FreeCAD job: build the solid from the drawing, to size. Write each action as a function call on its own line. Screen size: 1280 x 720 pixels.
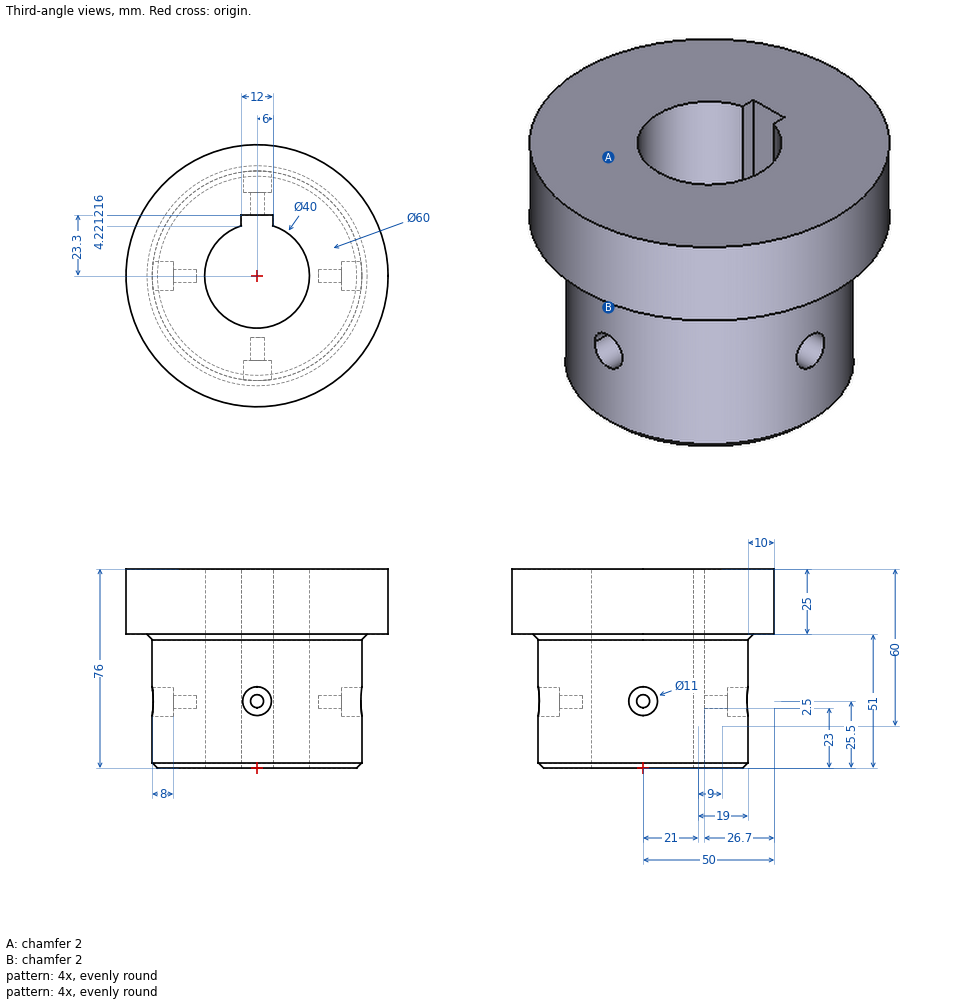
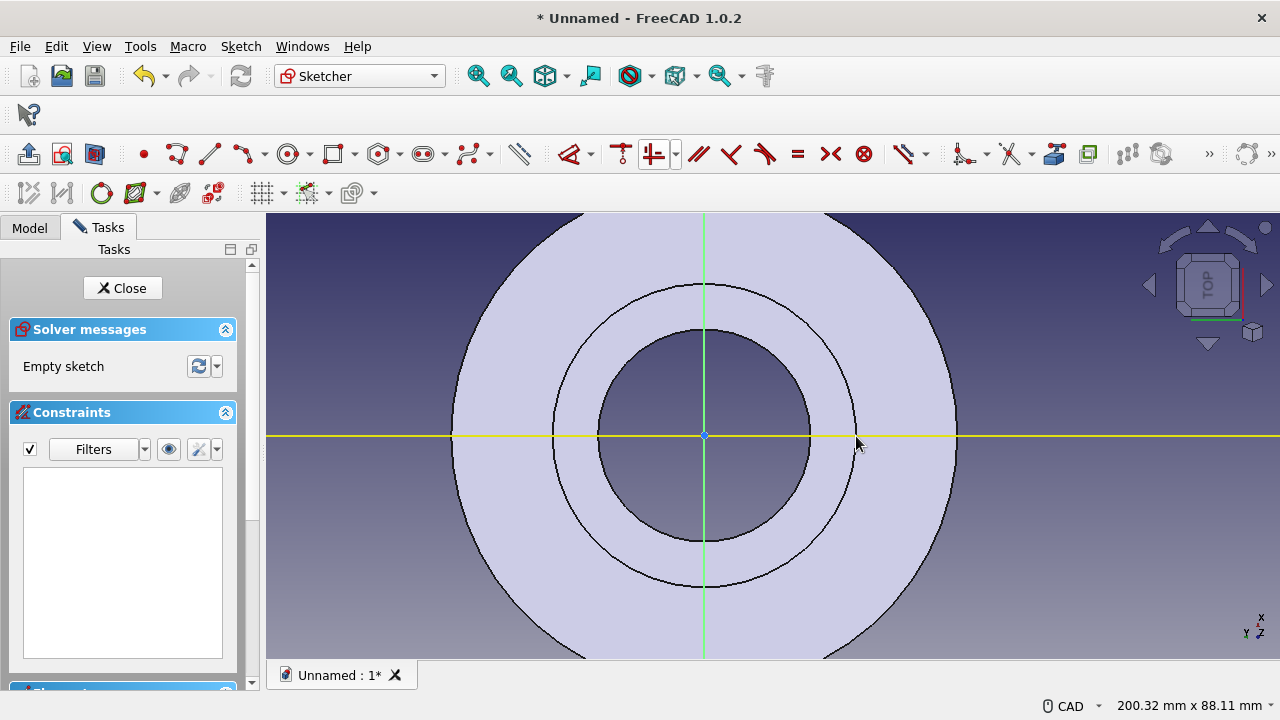
key(g)
key(c)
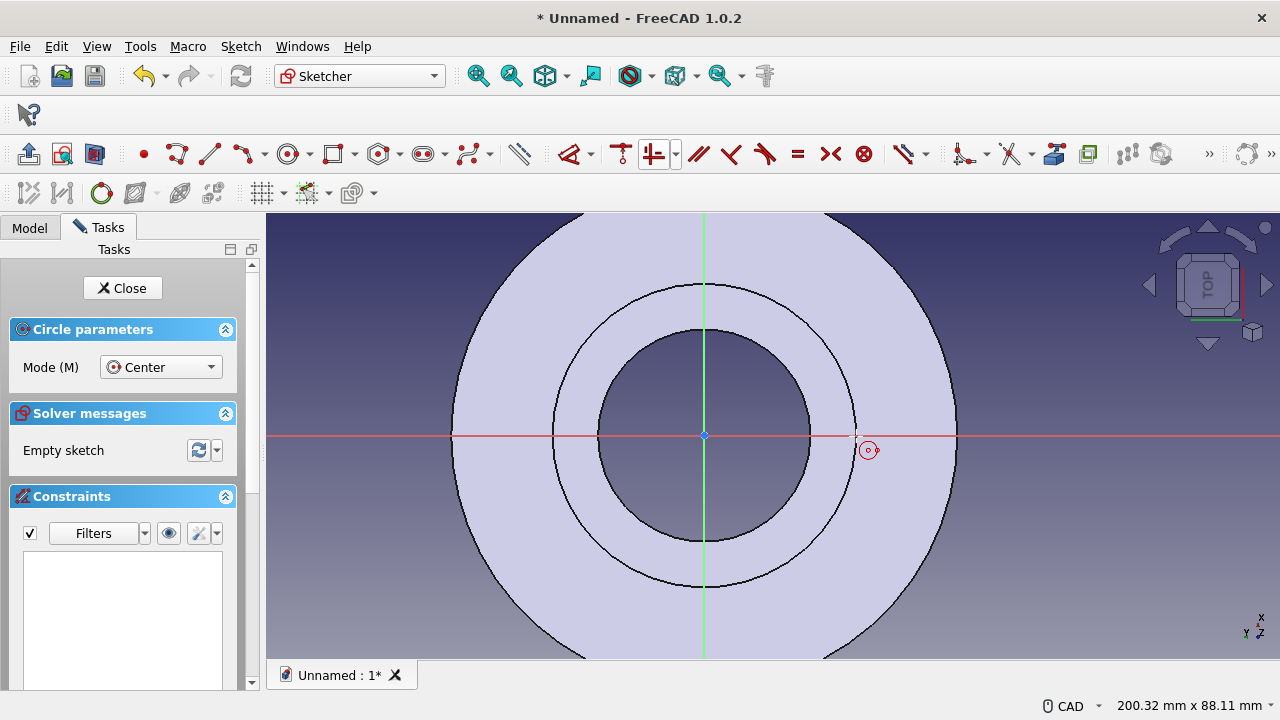
click(704, 436)
move(812, 328)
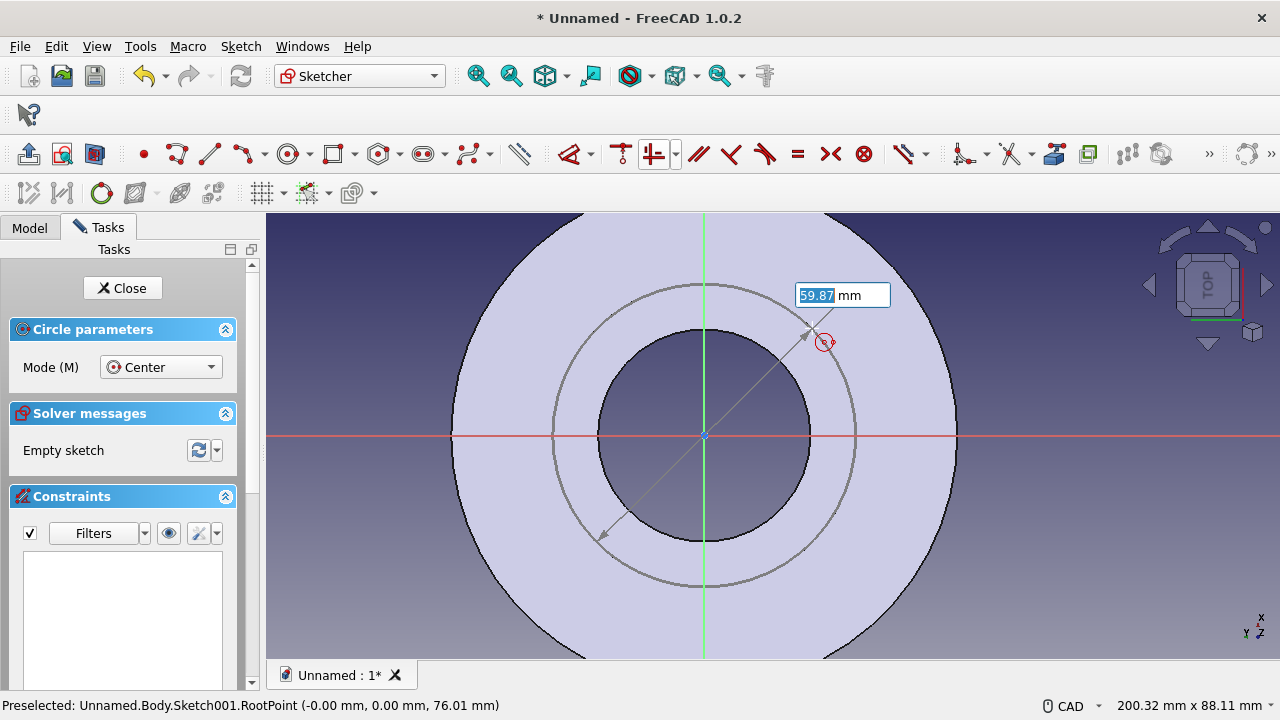
text(60)
key(Return)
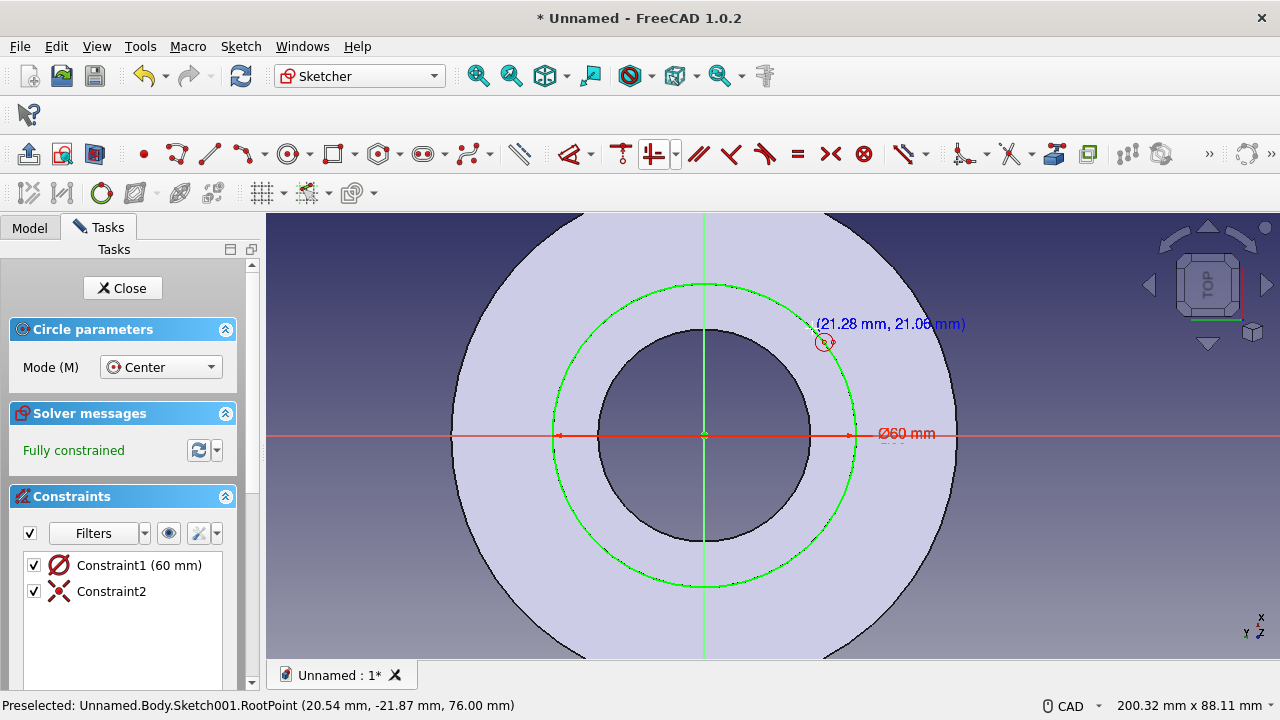
click(704, 436)
move(776, 364)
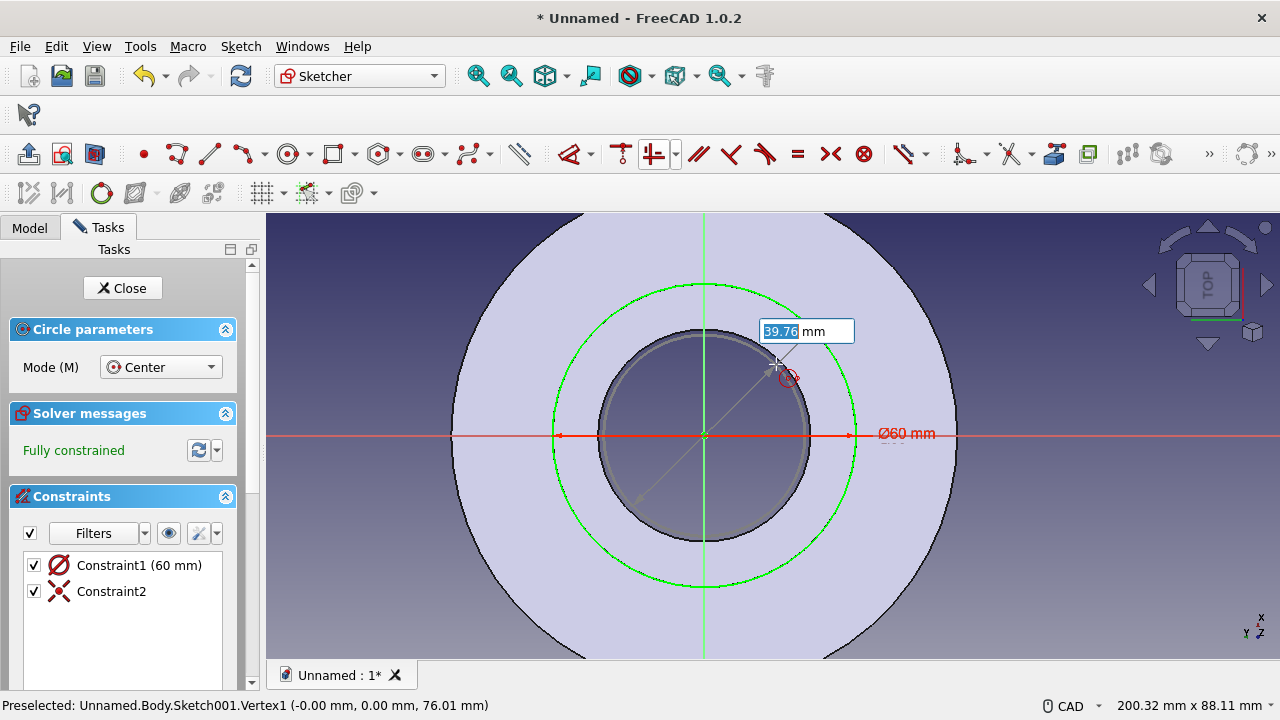
text(40)
key(Return)
key(Escape)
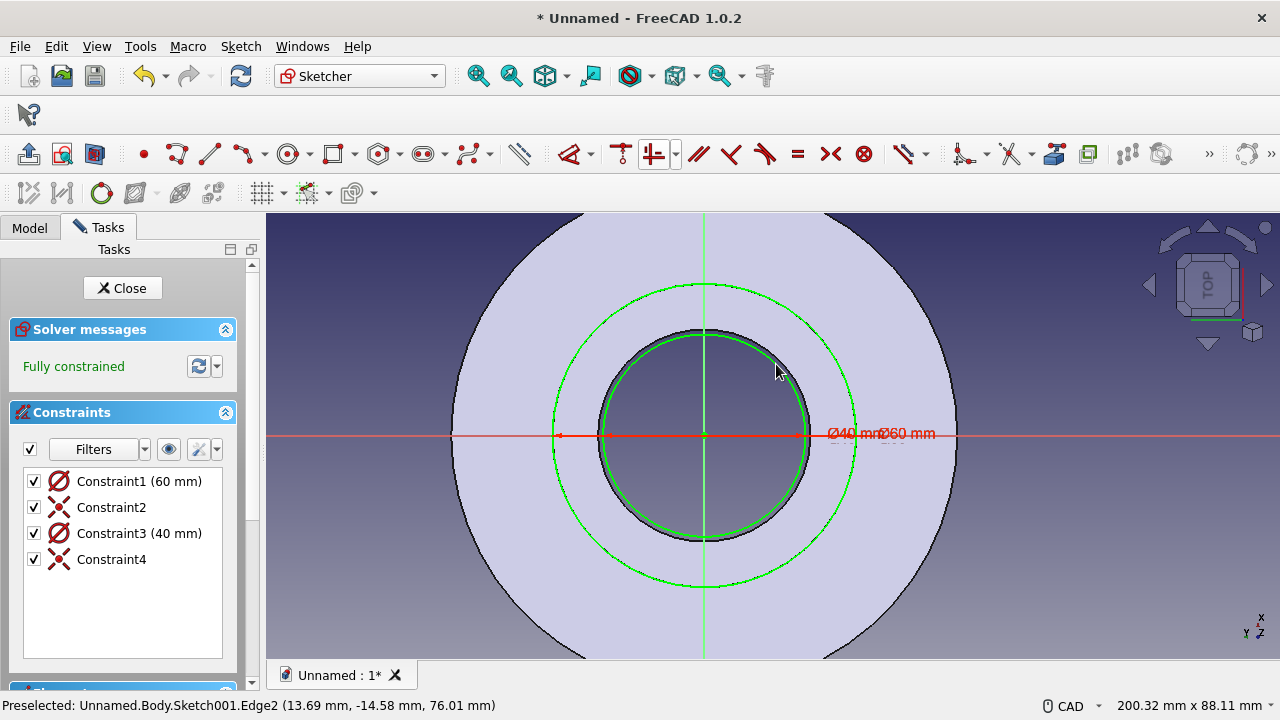
click(123, 288)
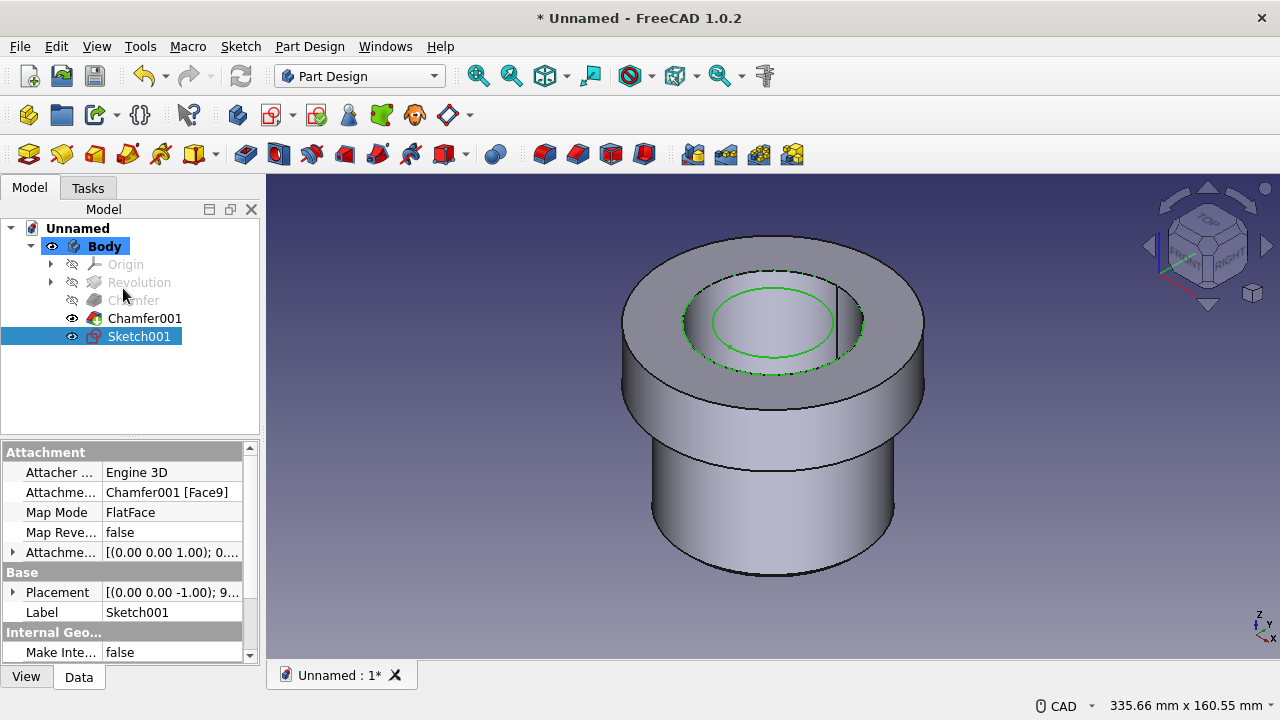
click(29, 154)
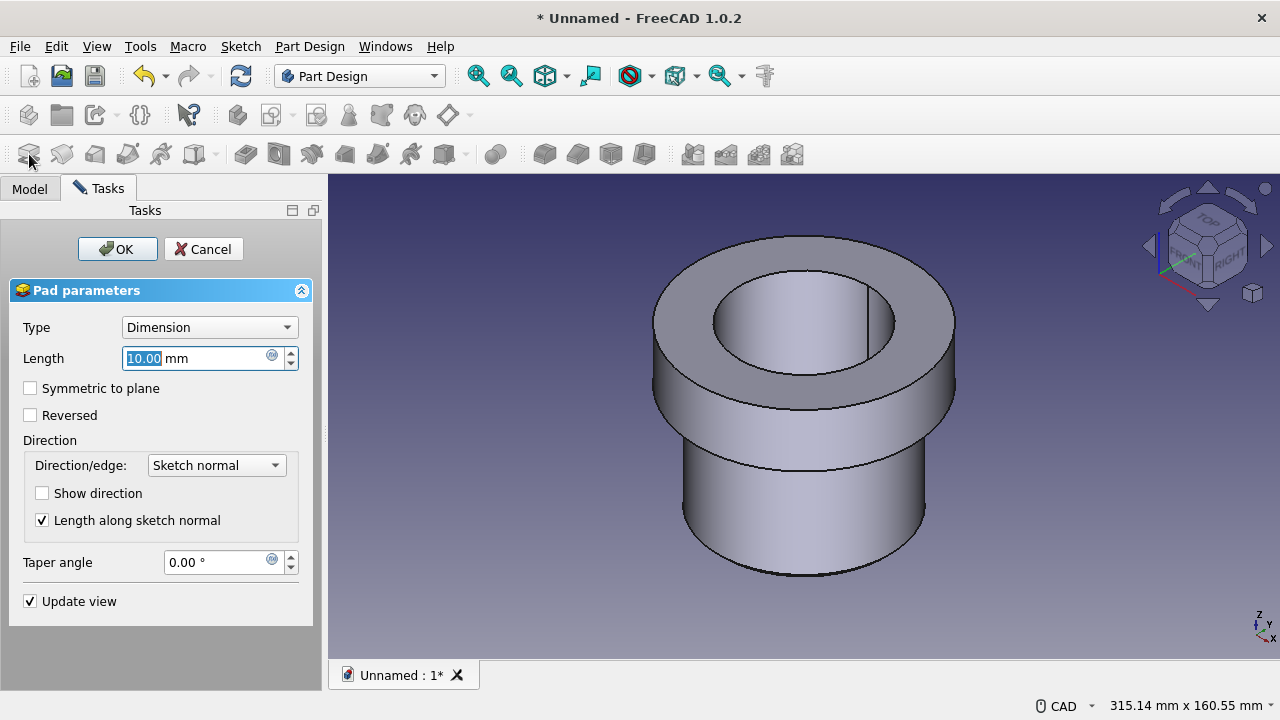
text(76)
key(Tab)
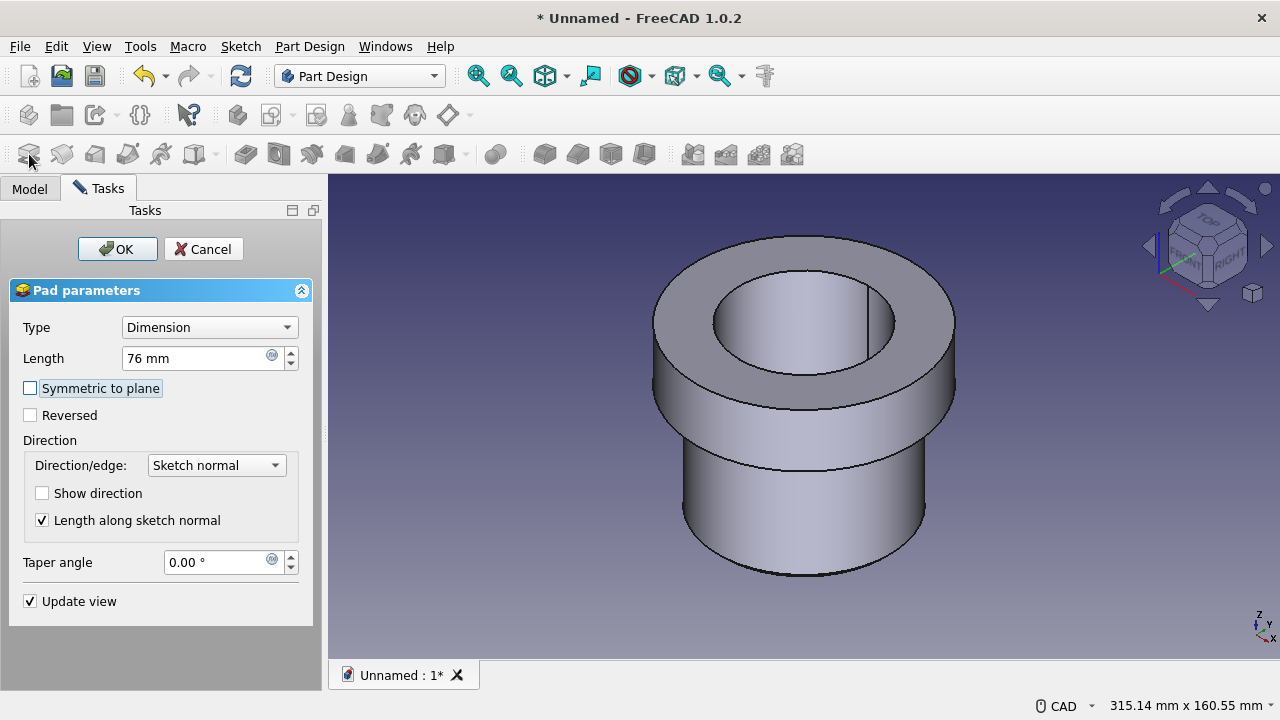
click(31, 415)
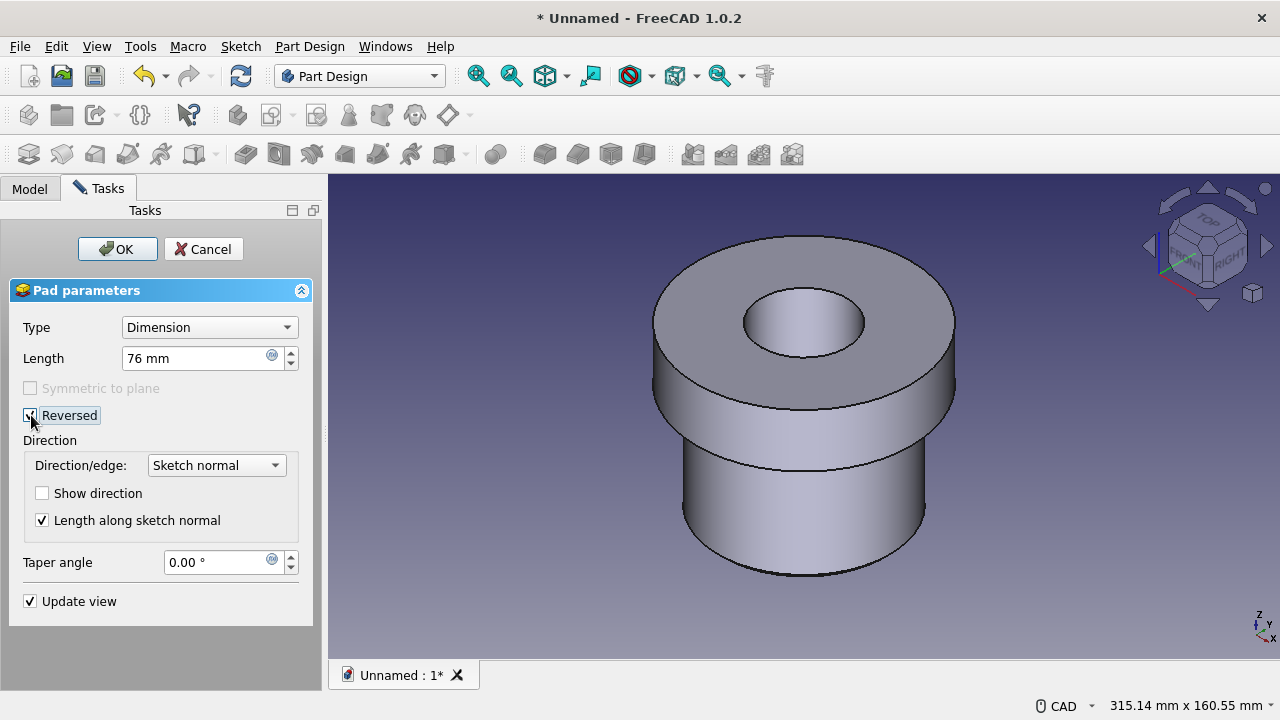
click(118, 249)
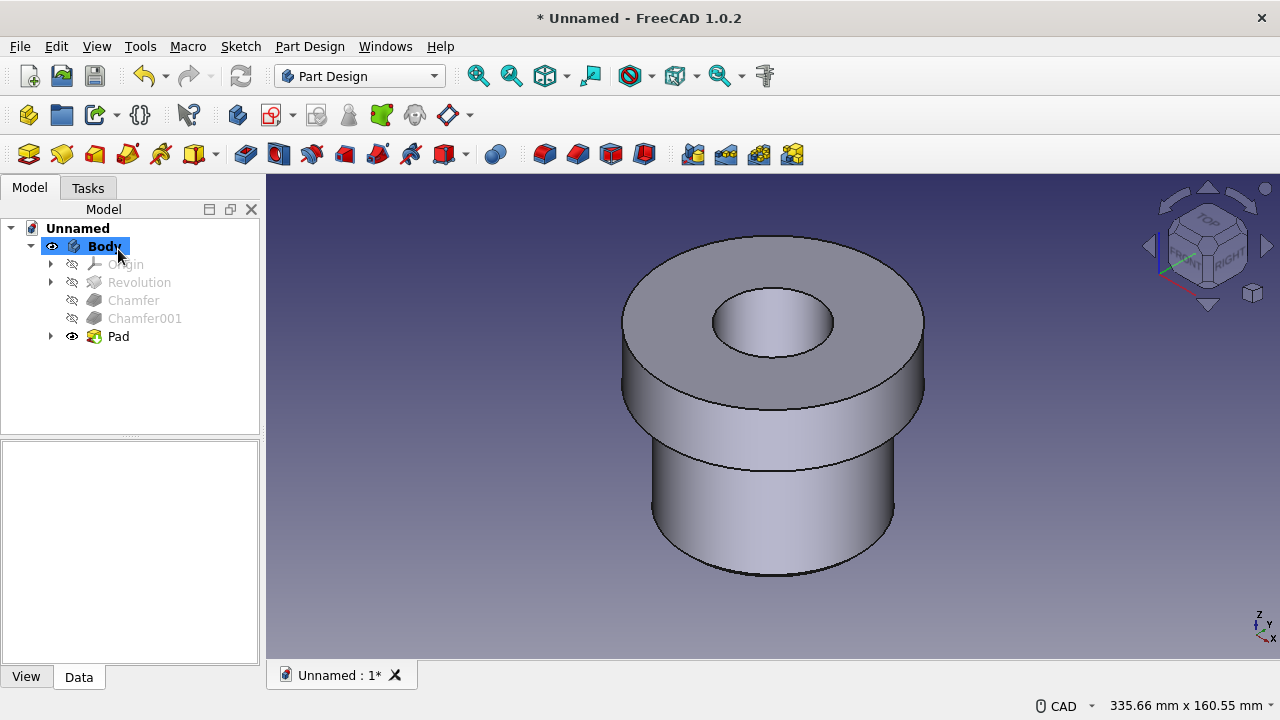
key(5)